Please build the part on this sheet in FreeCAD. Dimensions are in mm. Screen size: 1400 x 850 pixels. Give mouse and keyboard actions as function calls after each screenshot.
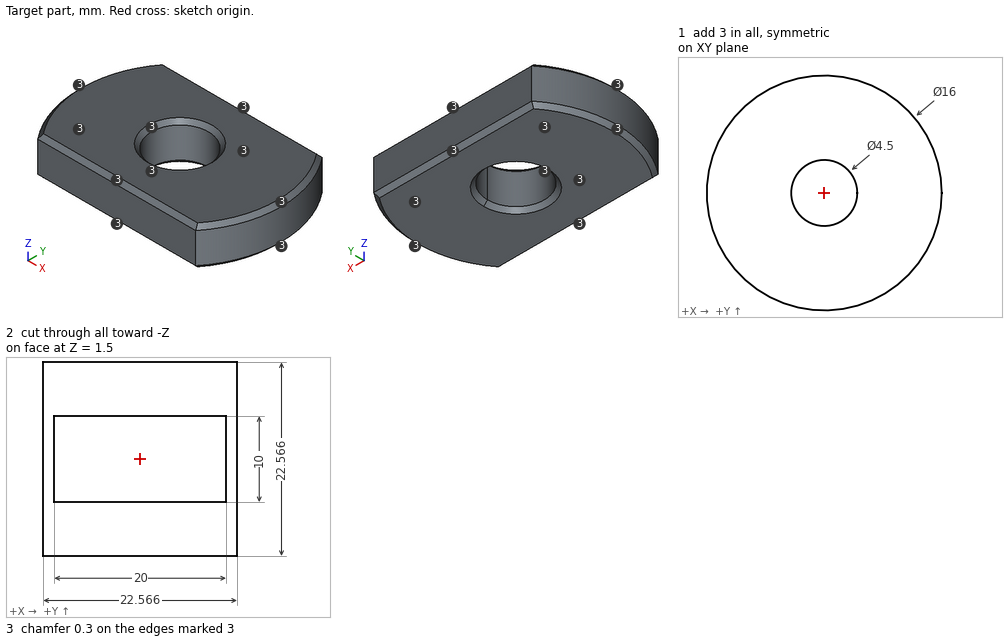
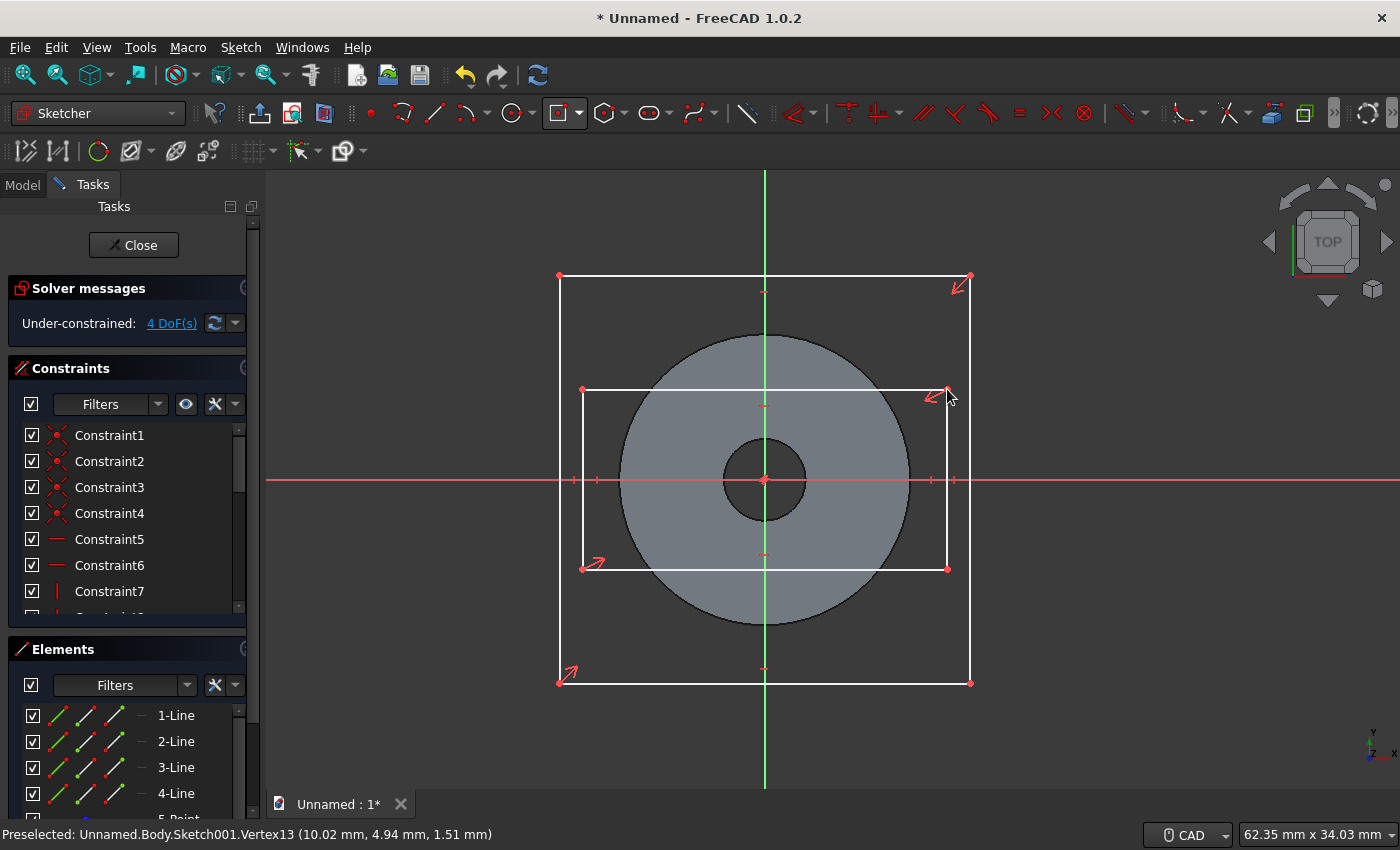
click(692, 570)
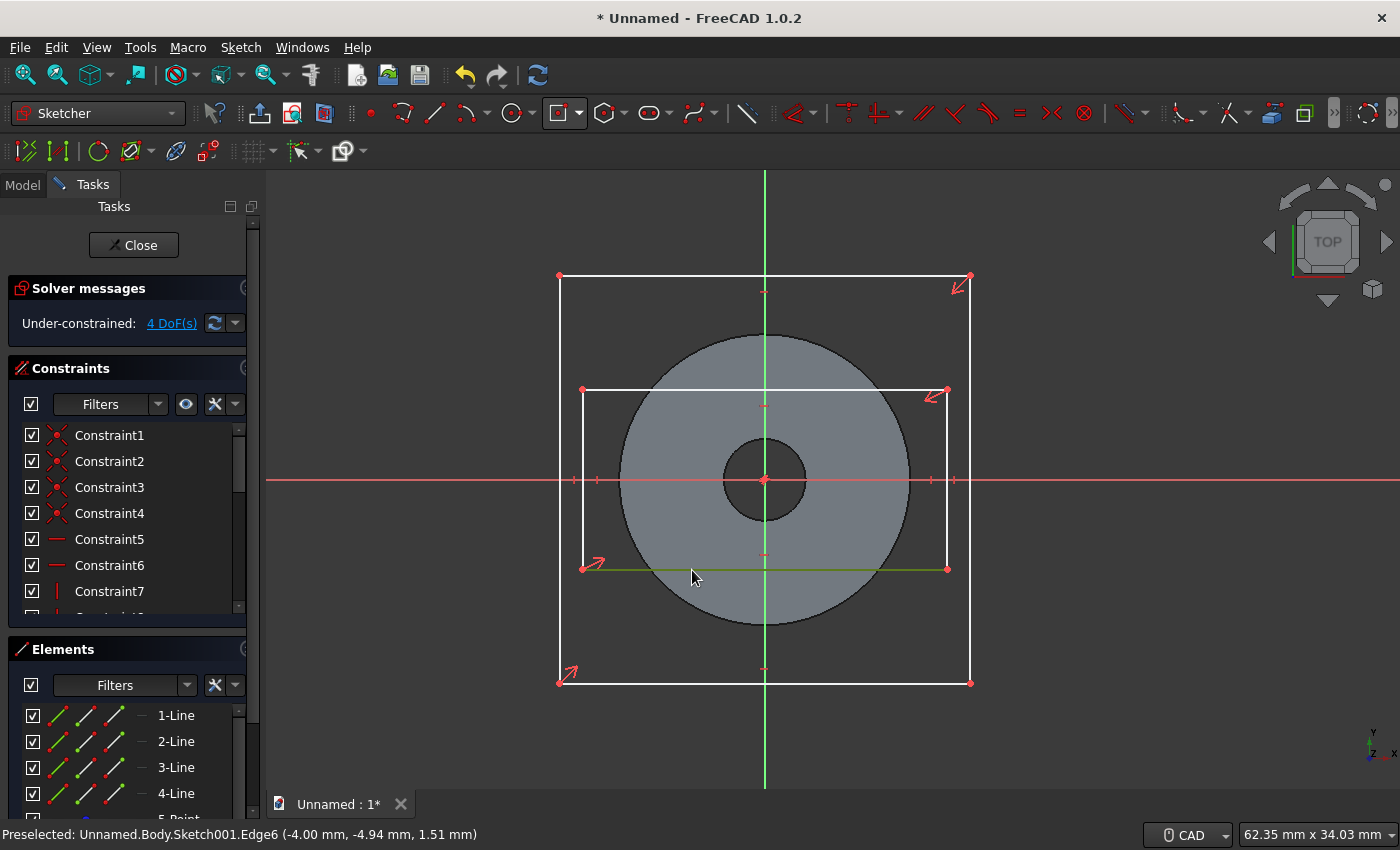
click(816, 114)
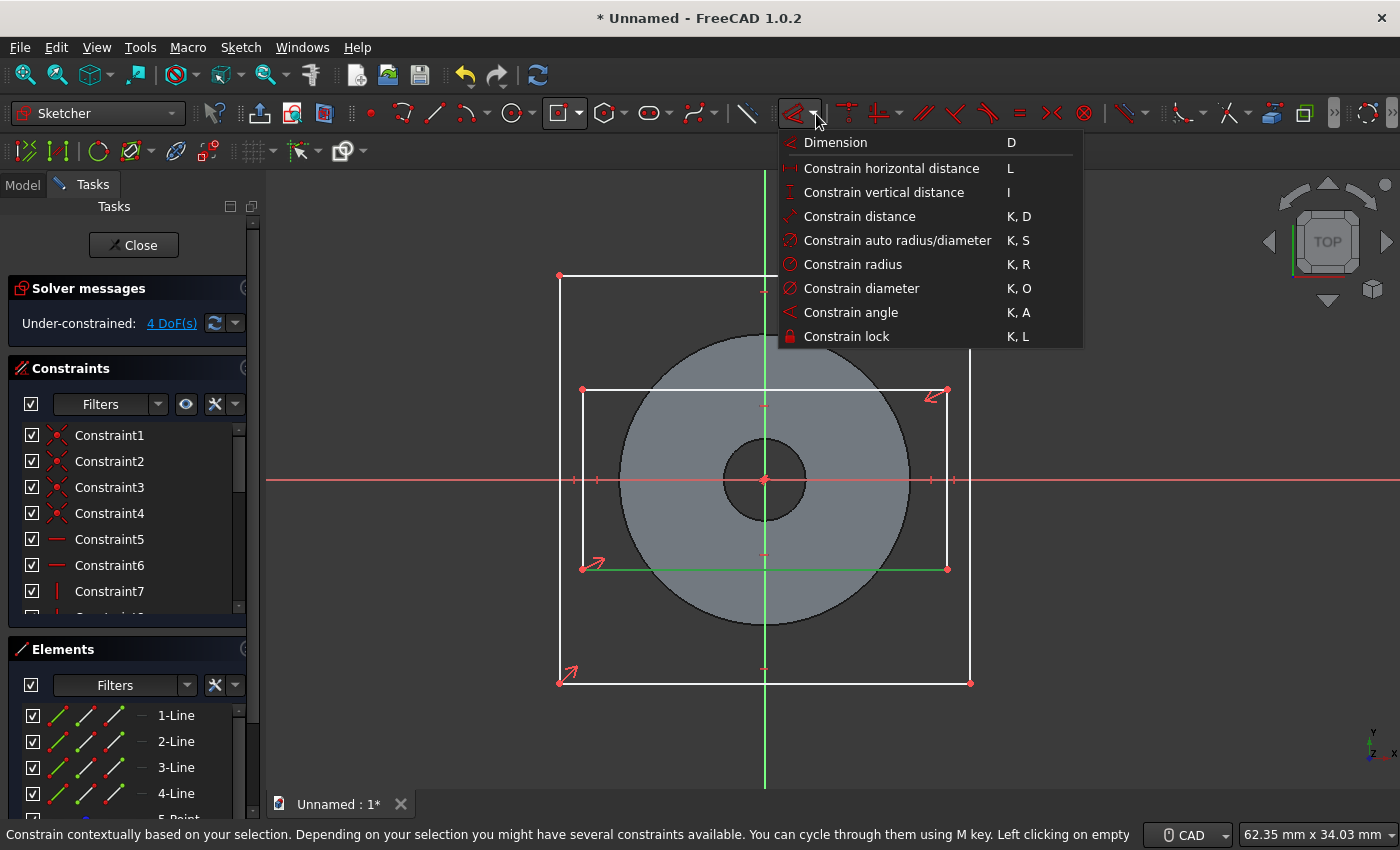
click(931, 168)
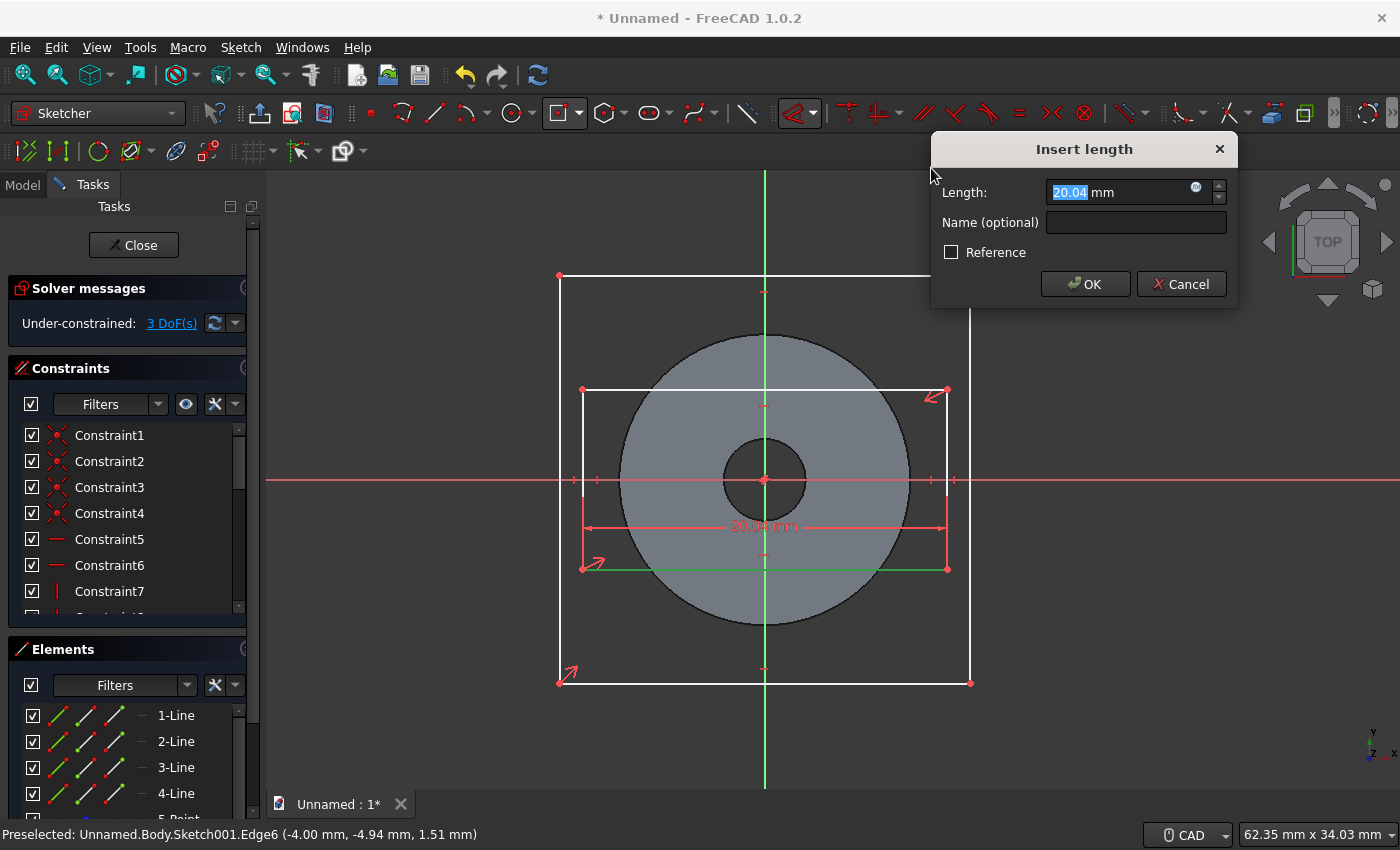
text(20)
key(Return)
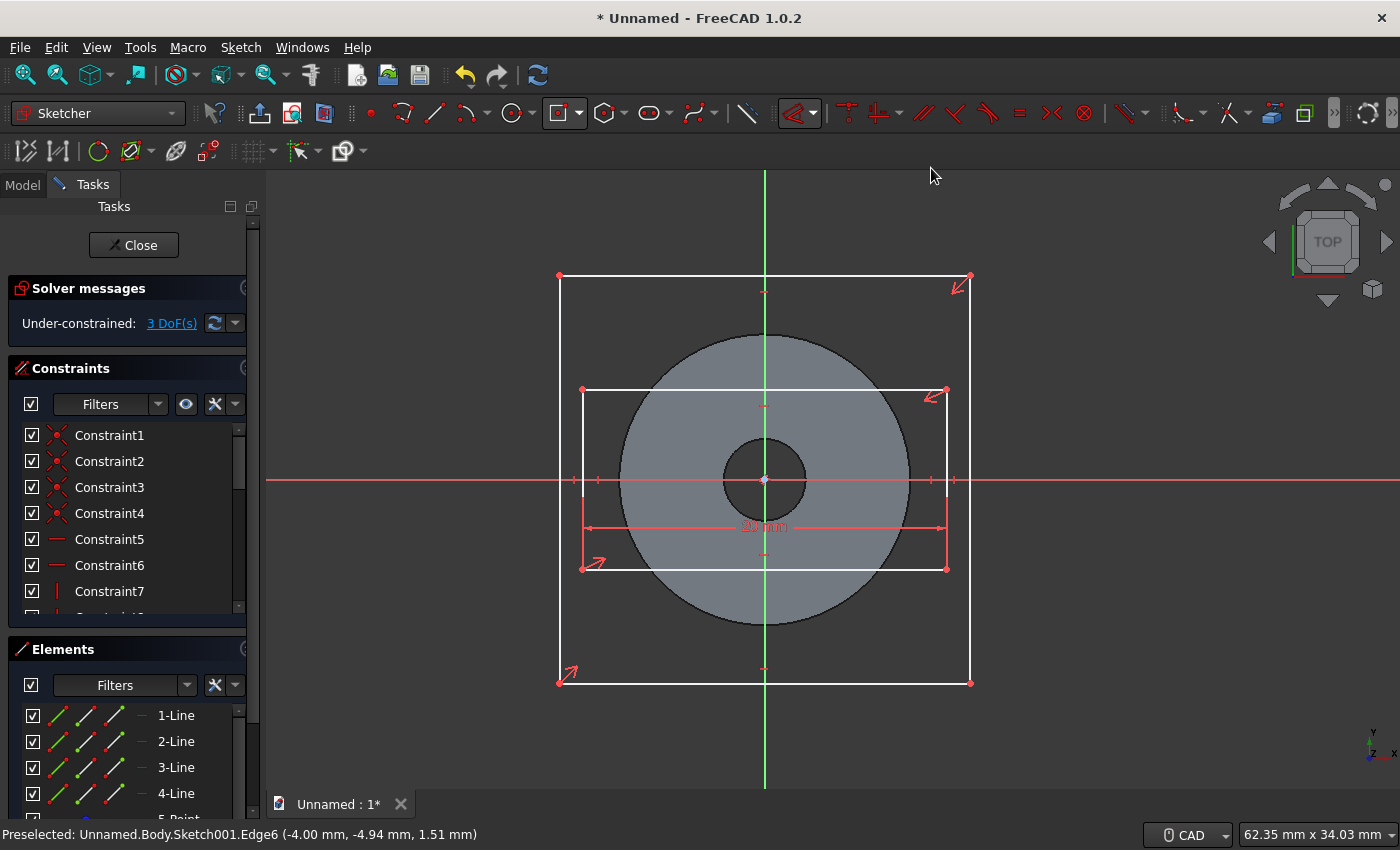
click(947, 516)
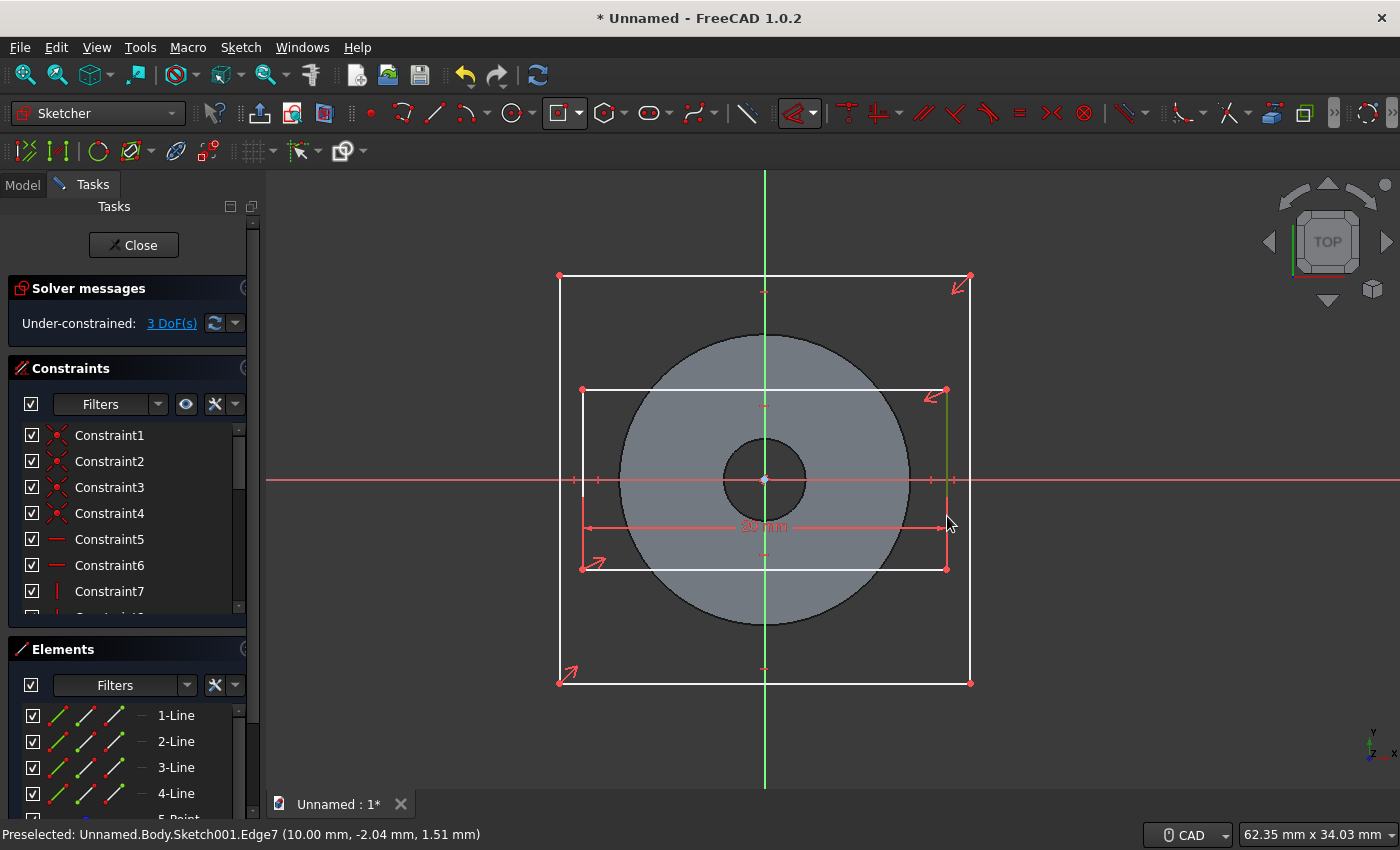
key(i)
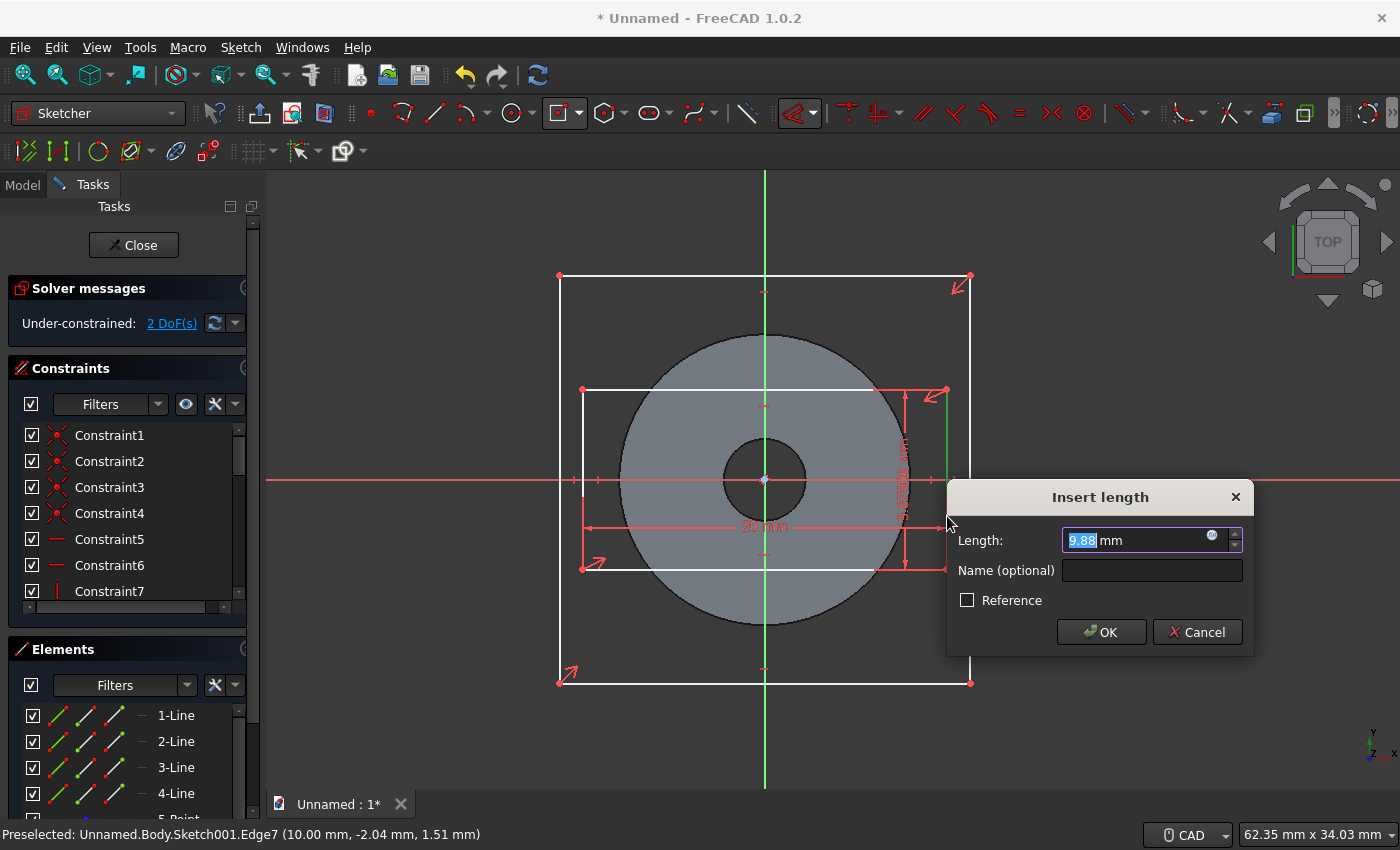
text(10)
key(Return)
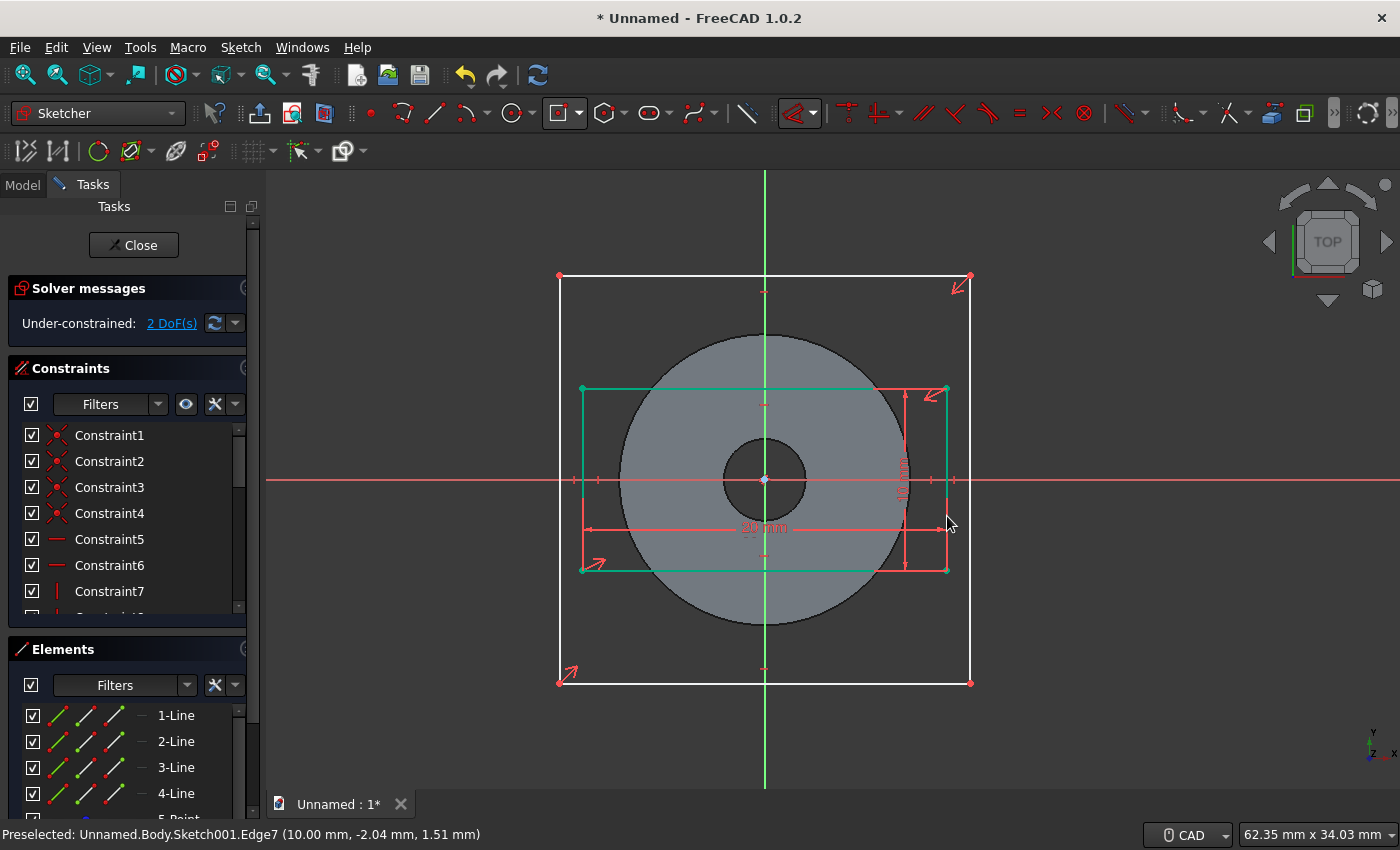
click(683, 684)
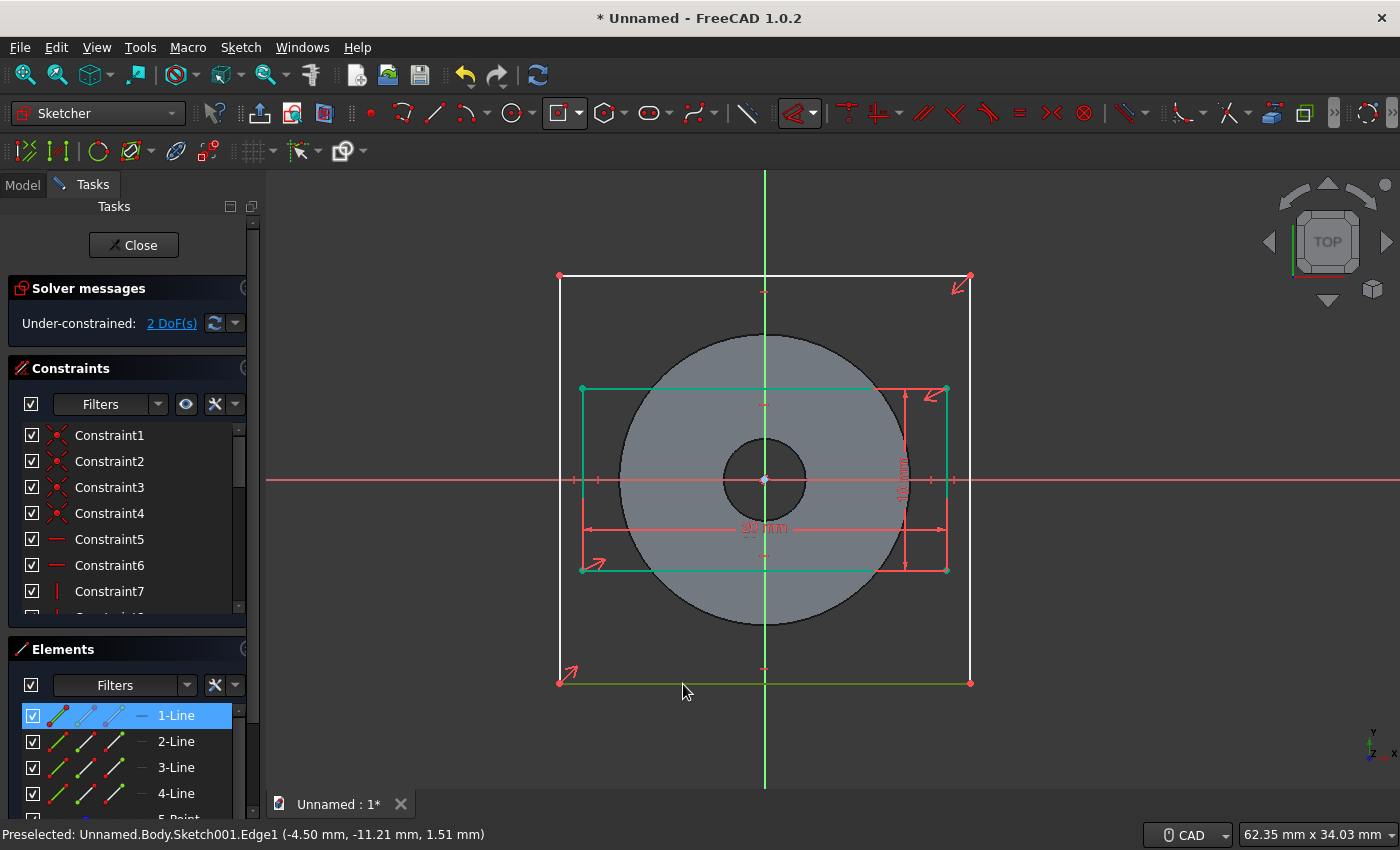
key(l)